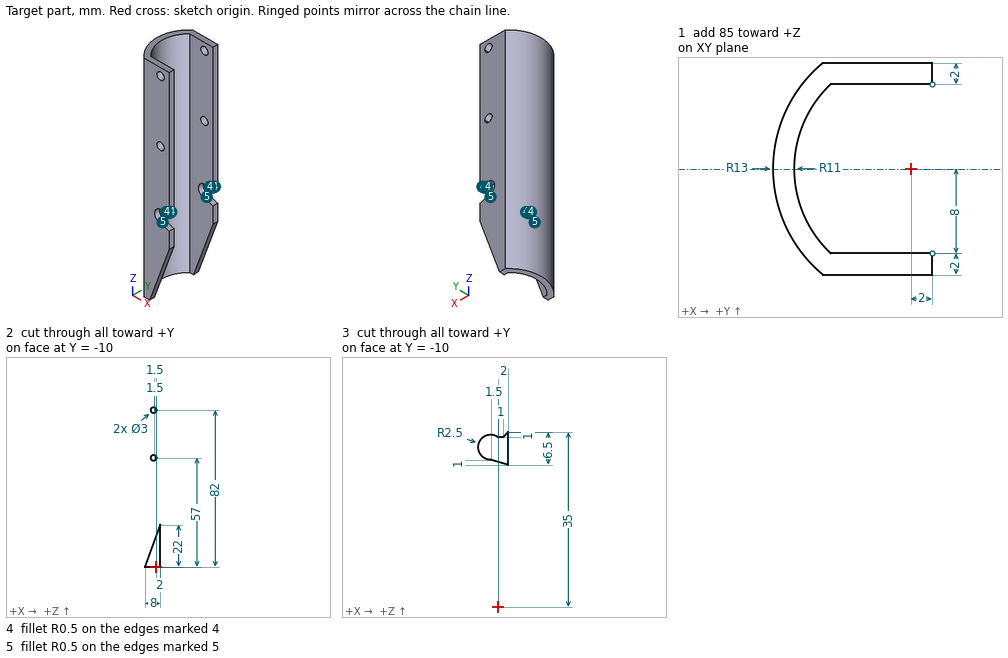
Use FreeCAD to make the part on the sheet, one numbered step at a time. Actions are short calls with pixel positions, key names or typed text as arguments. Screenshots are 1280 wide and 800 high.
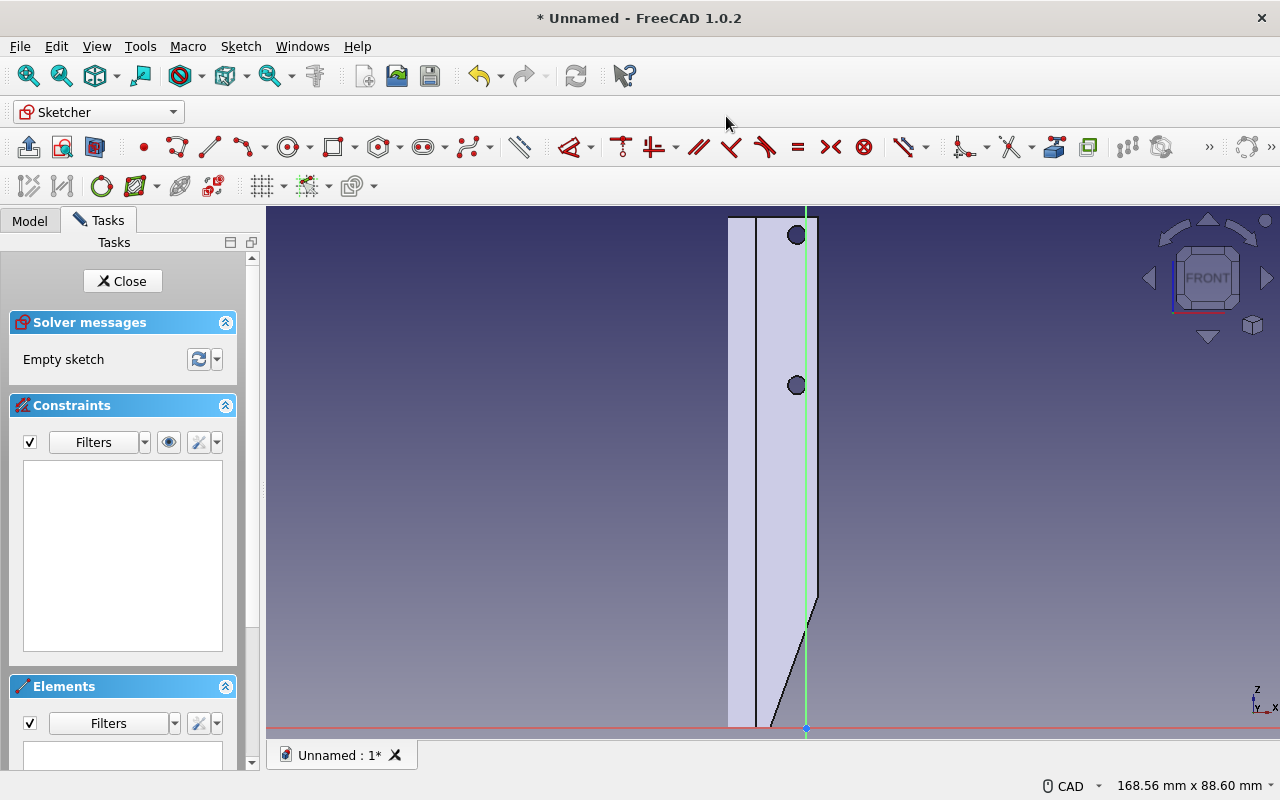
scroll(812, 545, up, 11)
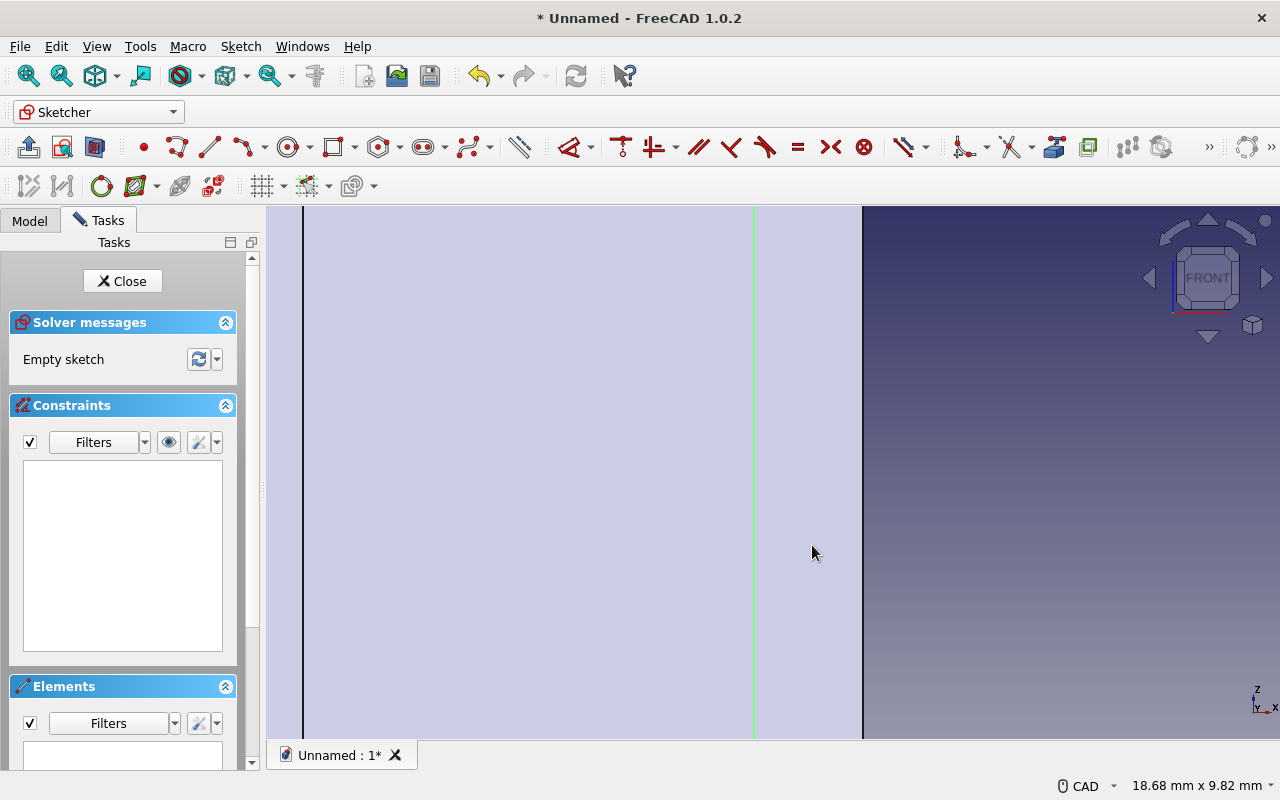
click(177, 148)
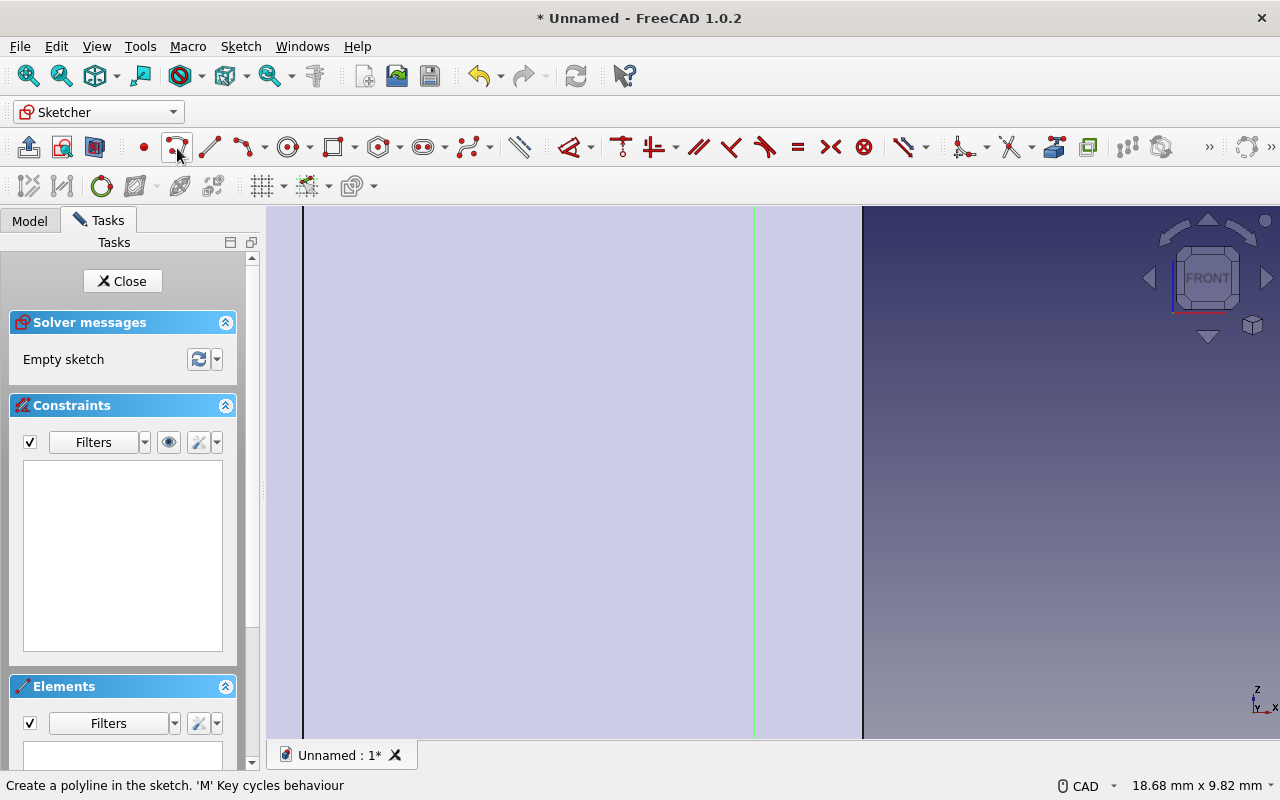
click(673, 591)
click(863, 646)
click(863, 293)
click(809, 347)
click(754, 347)
right_click(754, 347)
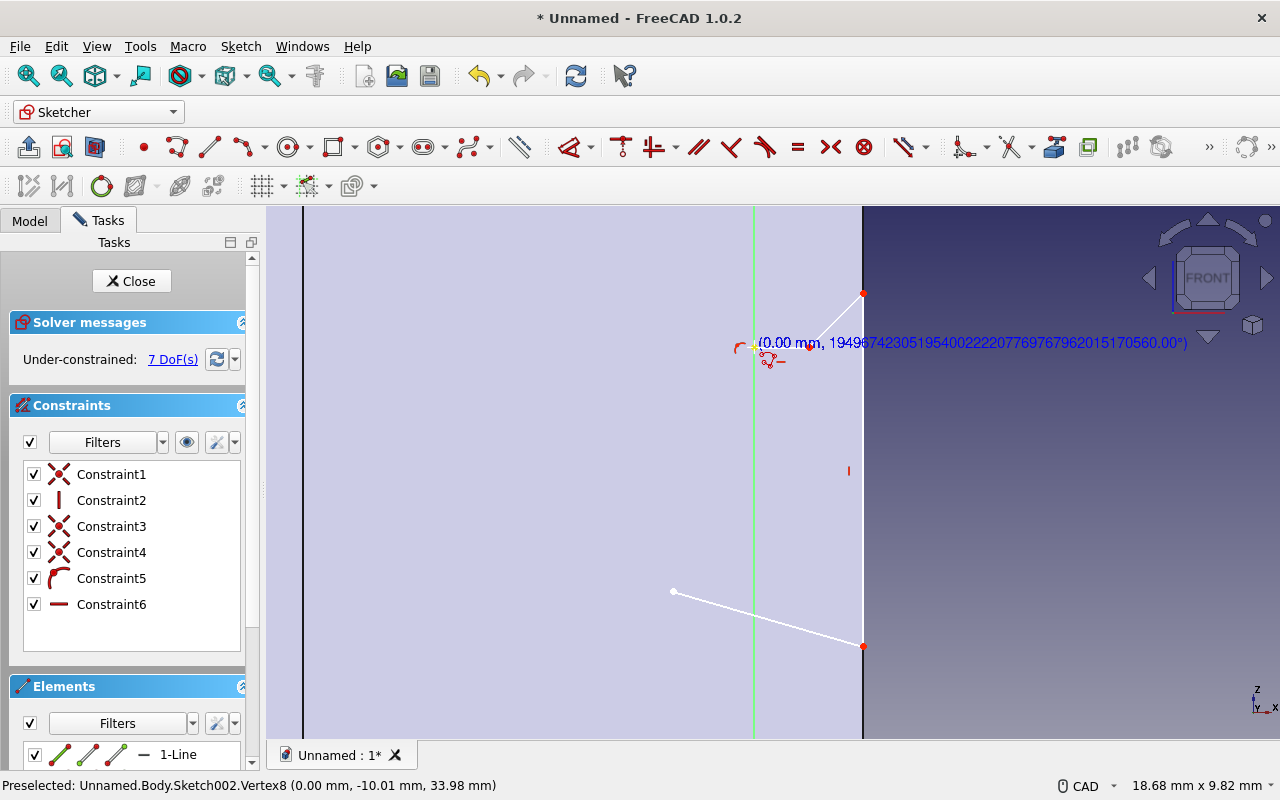
click(242, 148)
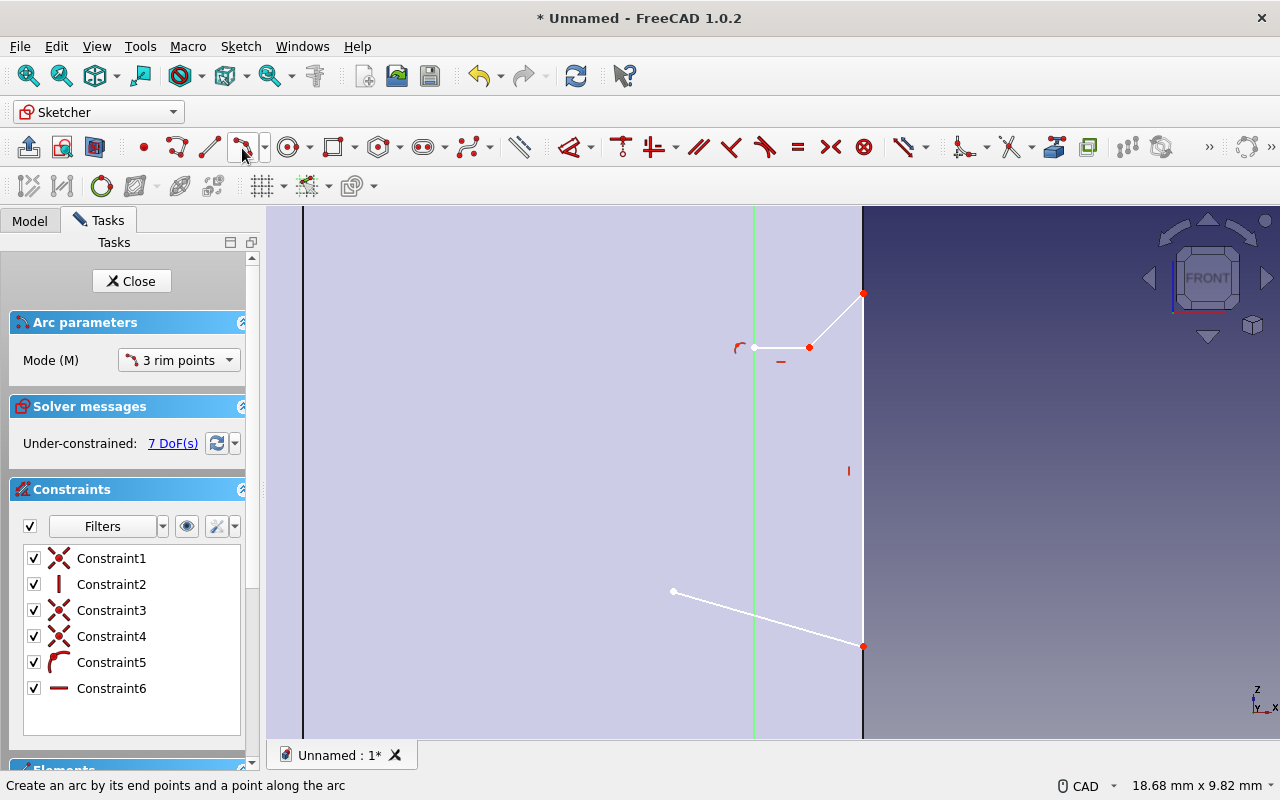
click(754, 348)
click(673, 592)
click(544, 413)
key(Escape)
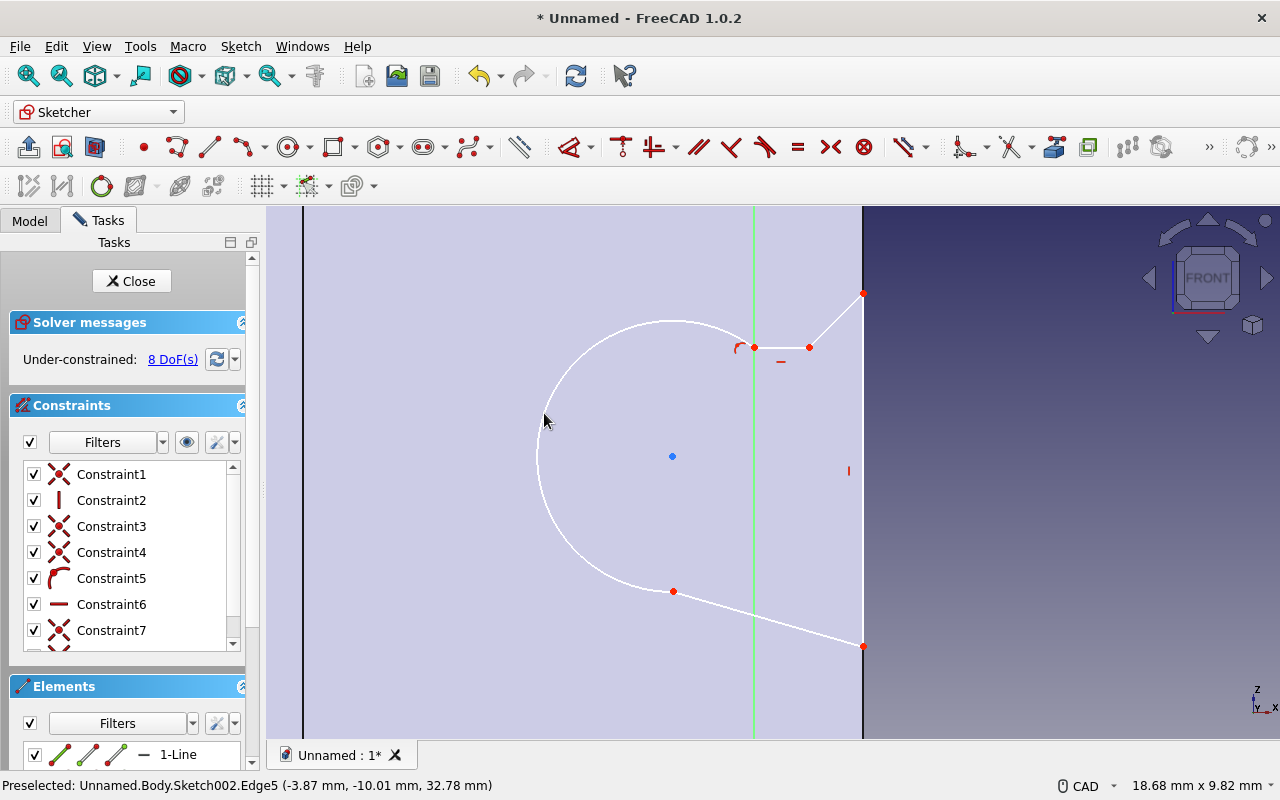
click(568, 148)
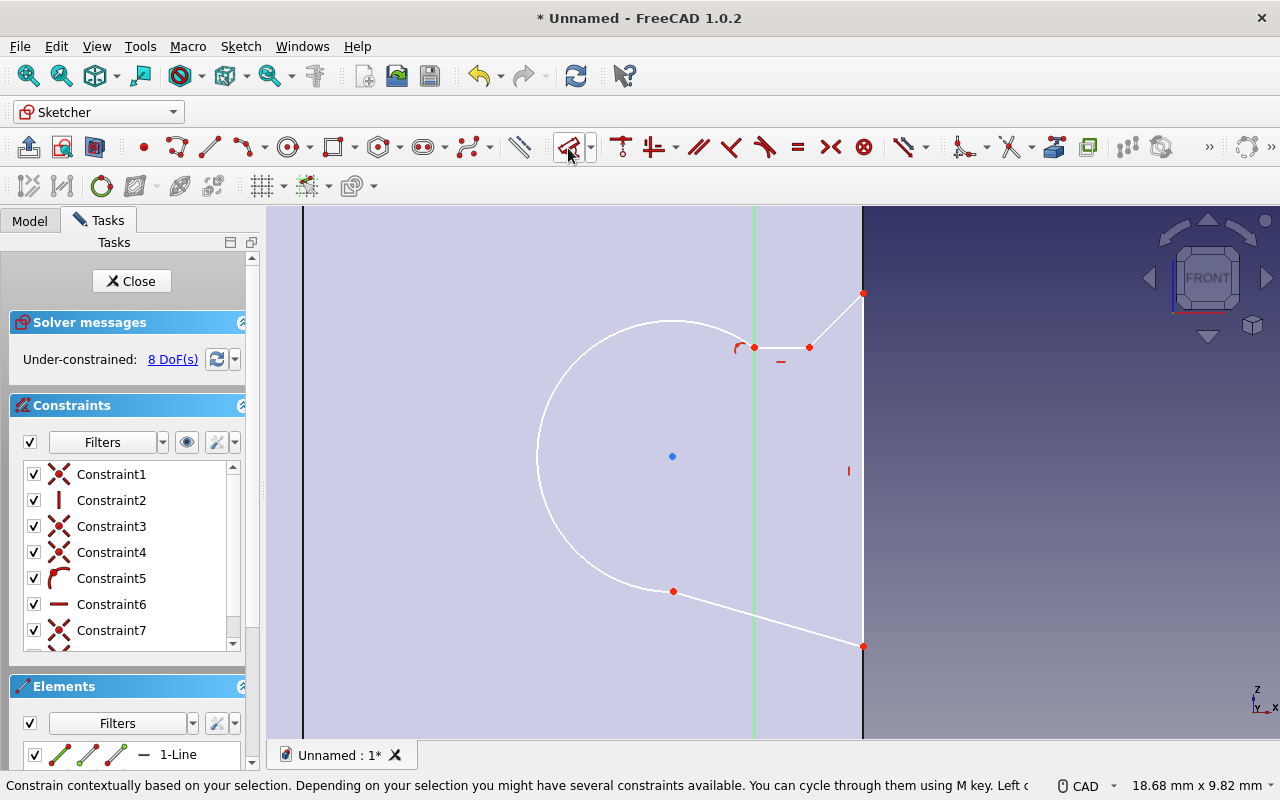
click(609, 337)
click(594, 309)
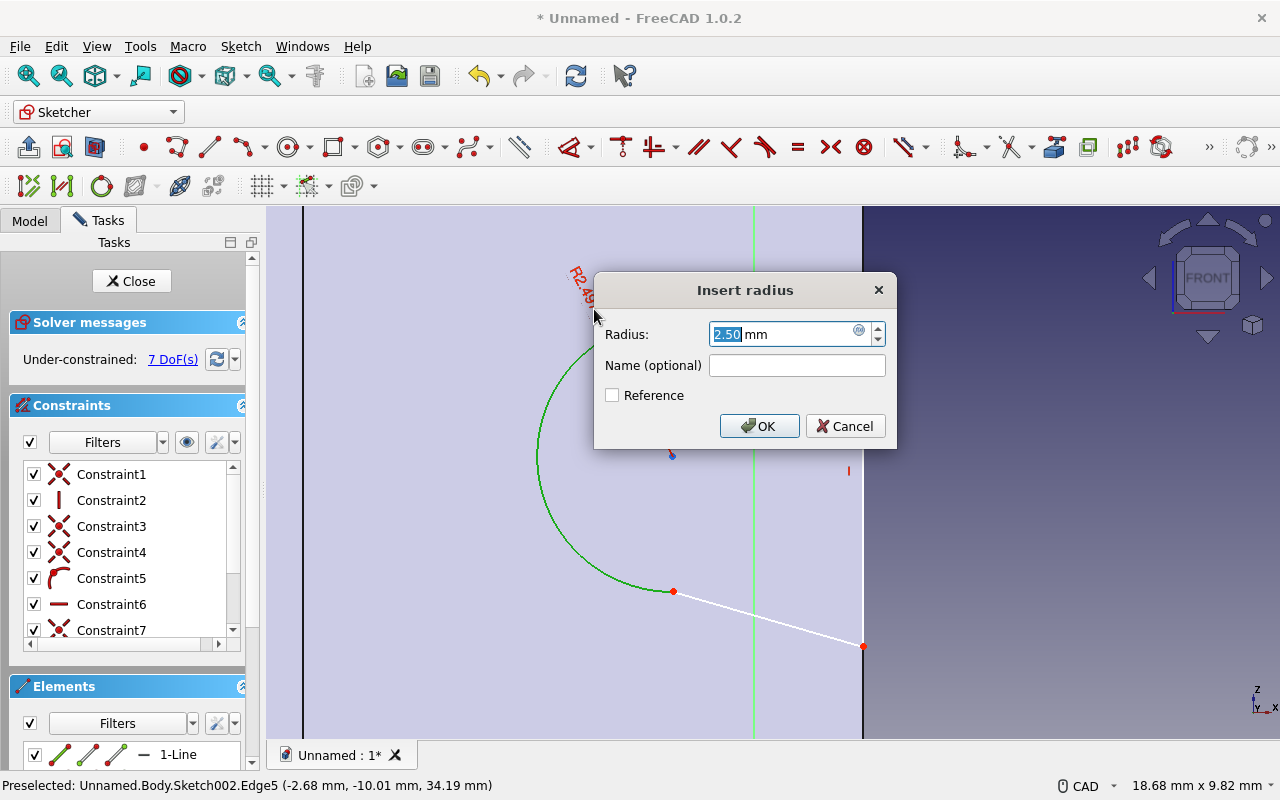
text(2.5)
key(Return)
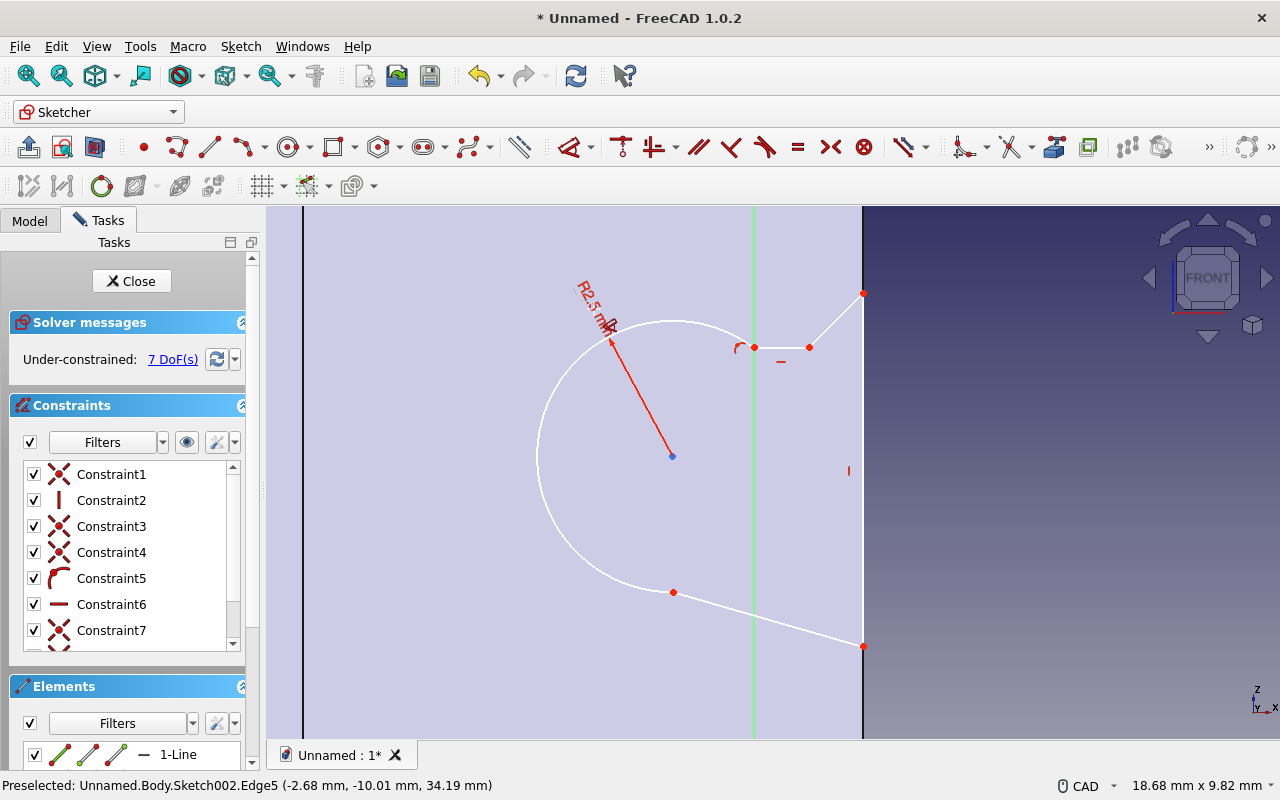
click(793, 348)
click(782, 314)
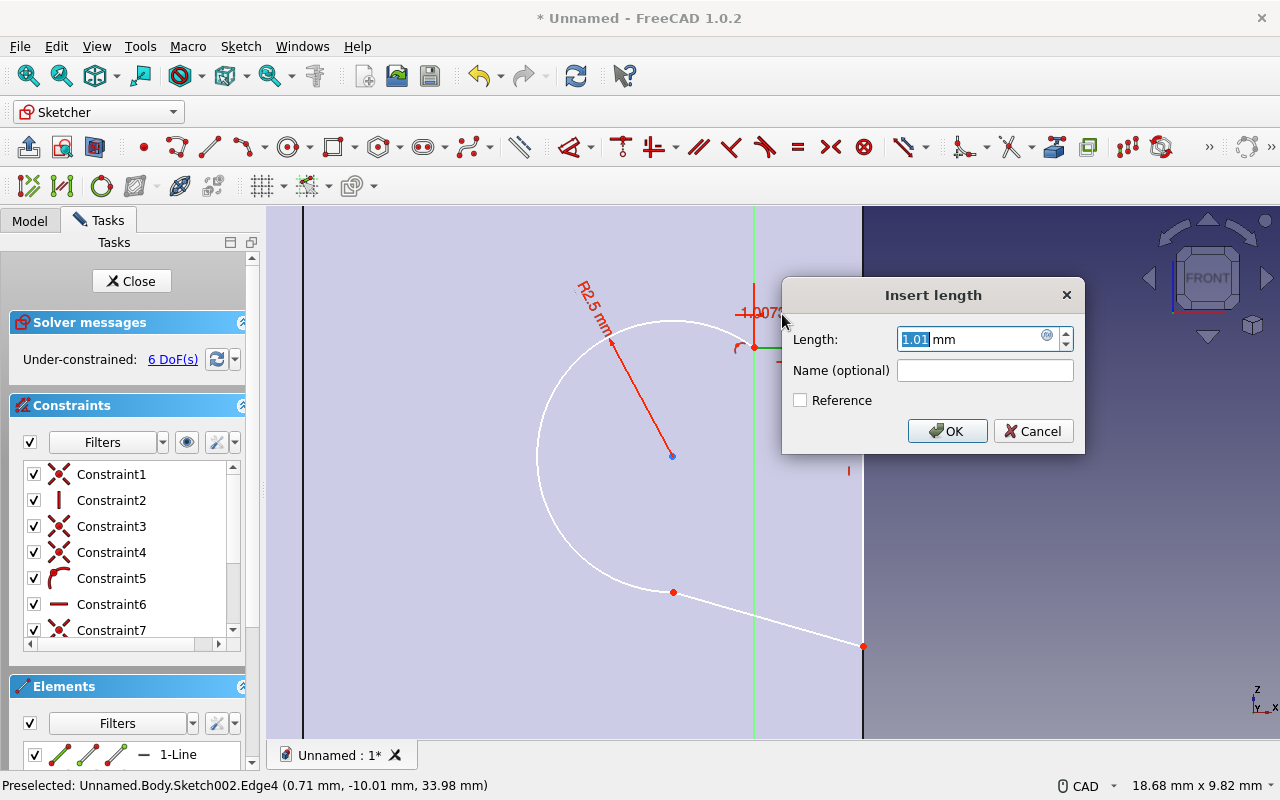
text(1)
key(Return)